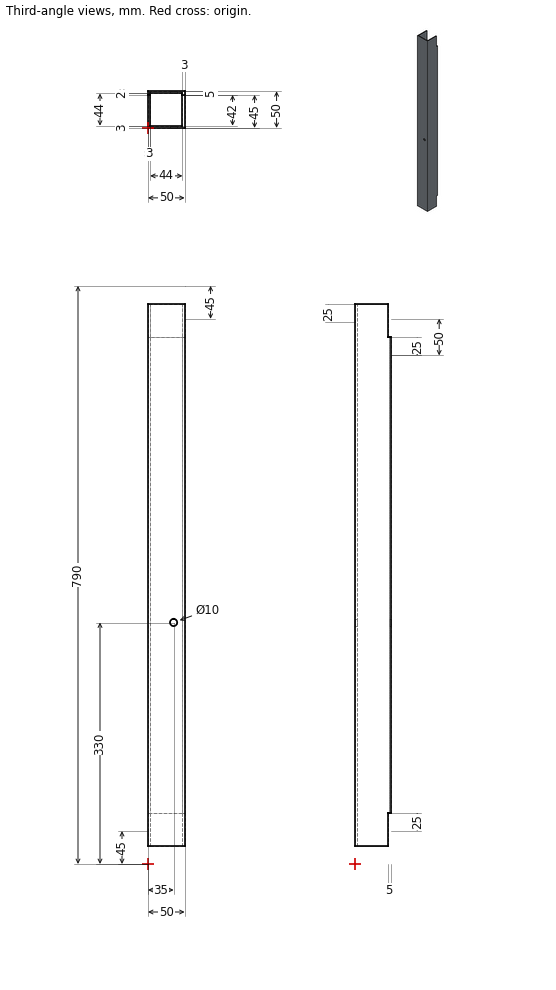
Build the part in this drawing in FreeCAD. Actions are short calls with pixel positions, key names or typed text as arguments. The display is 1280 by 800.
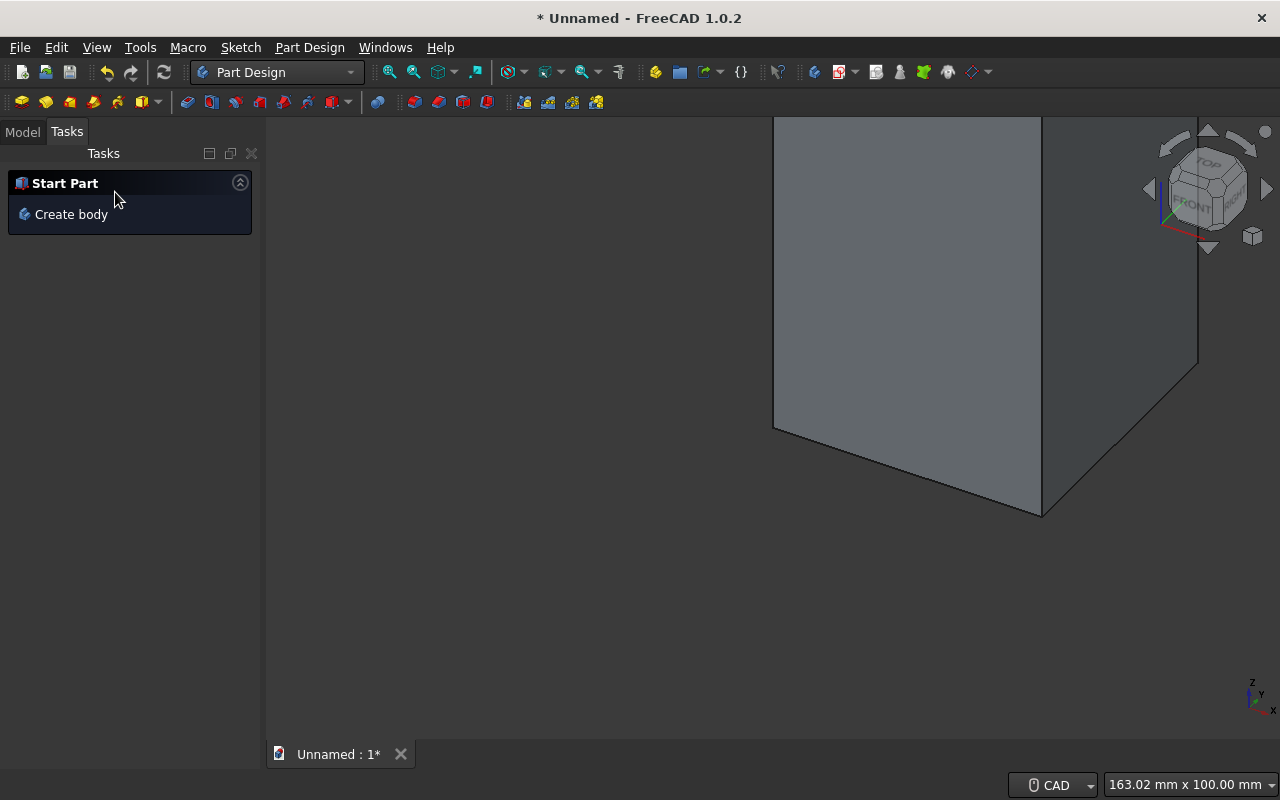
click(390, 72)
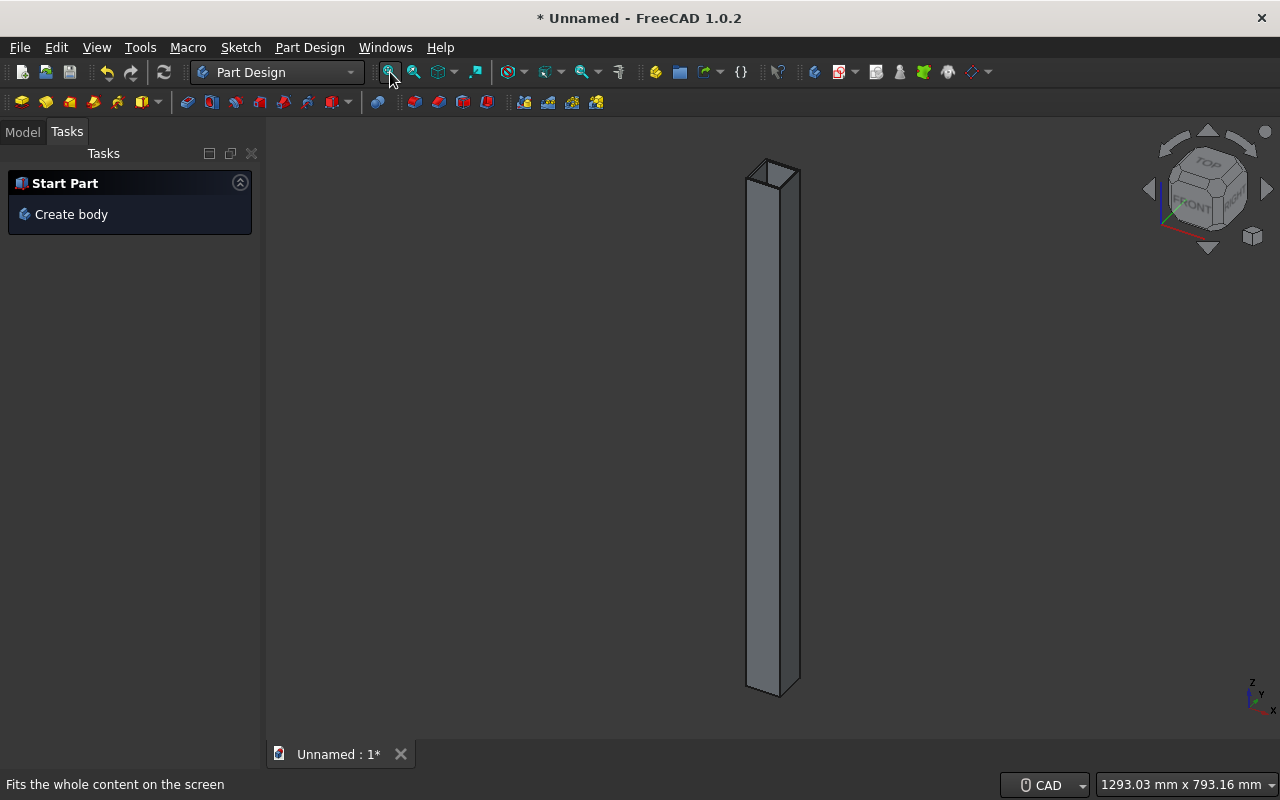
key(4)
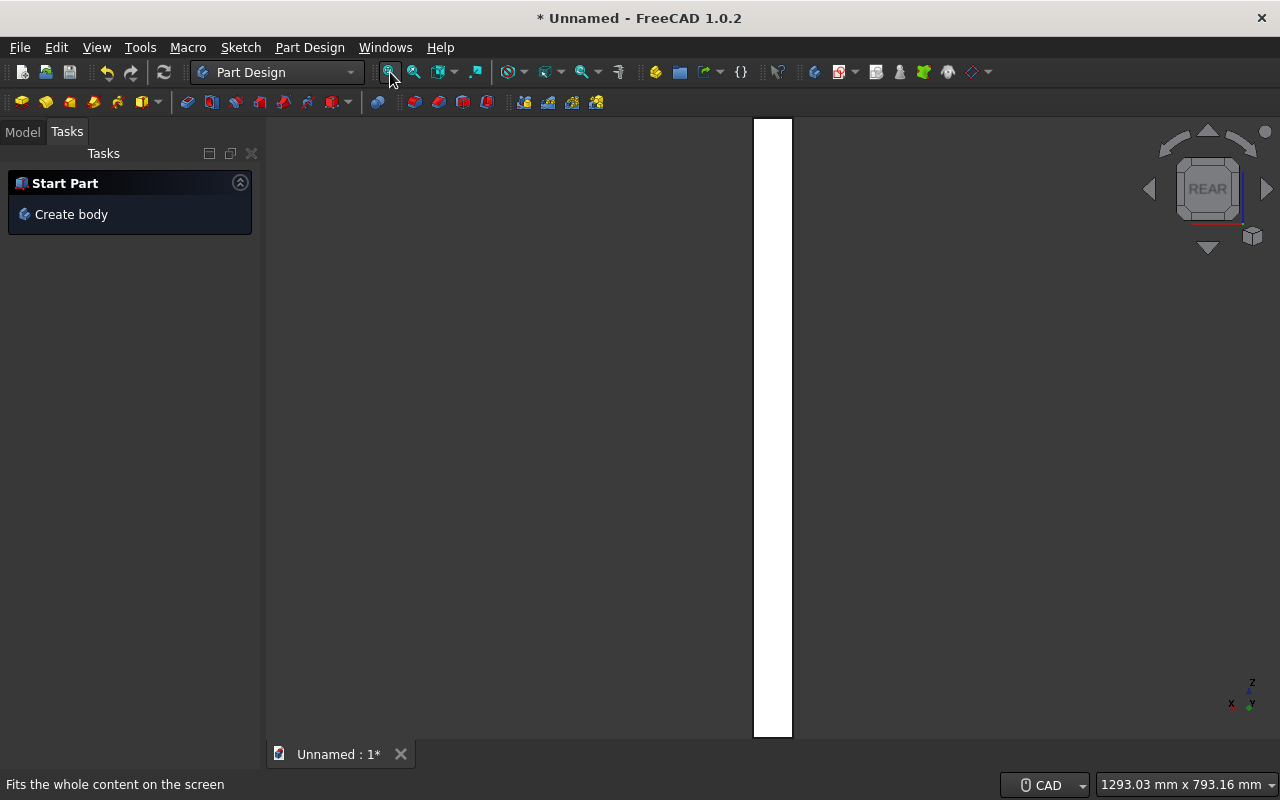
click(773, 161)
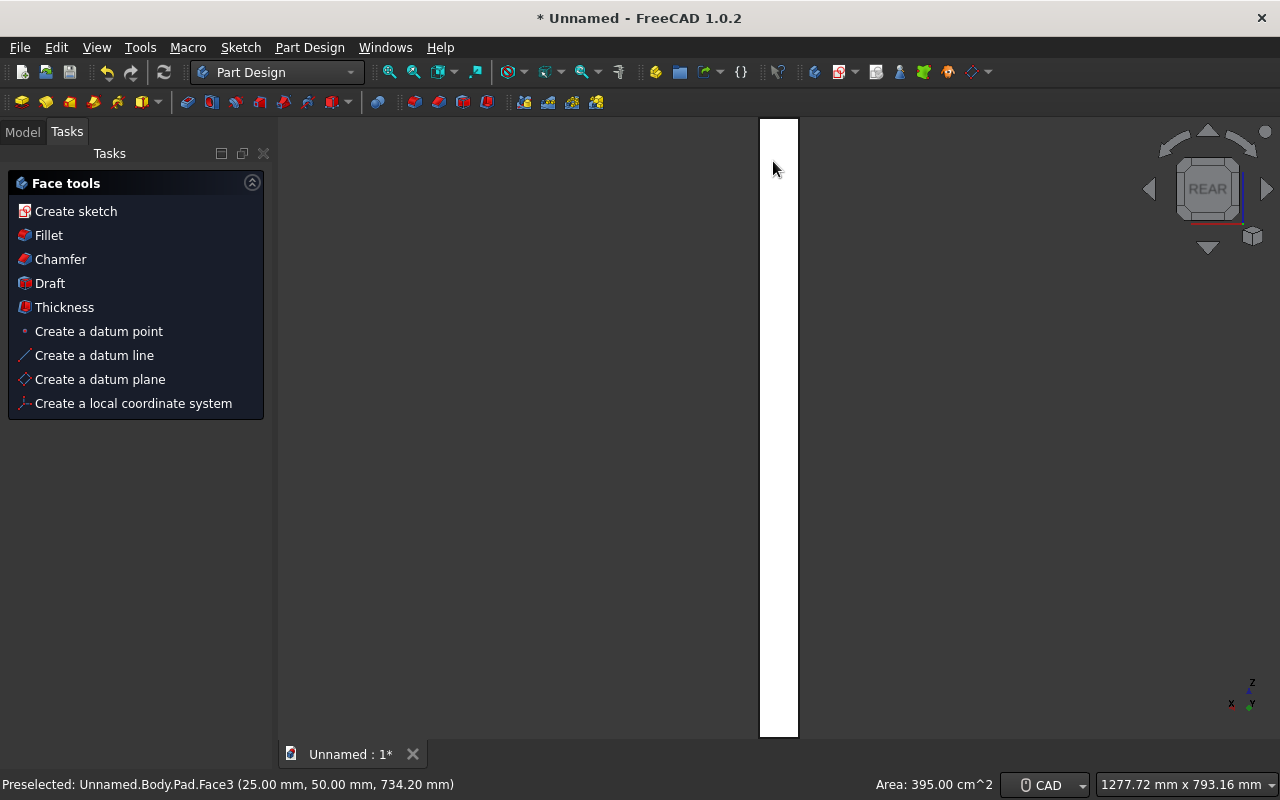
click(840, 72)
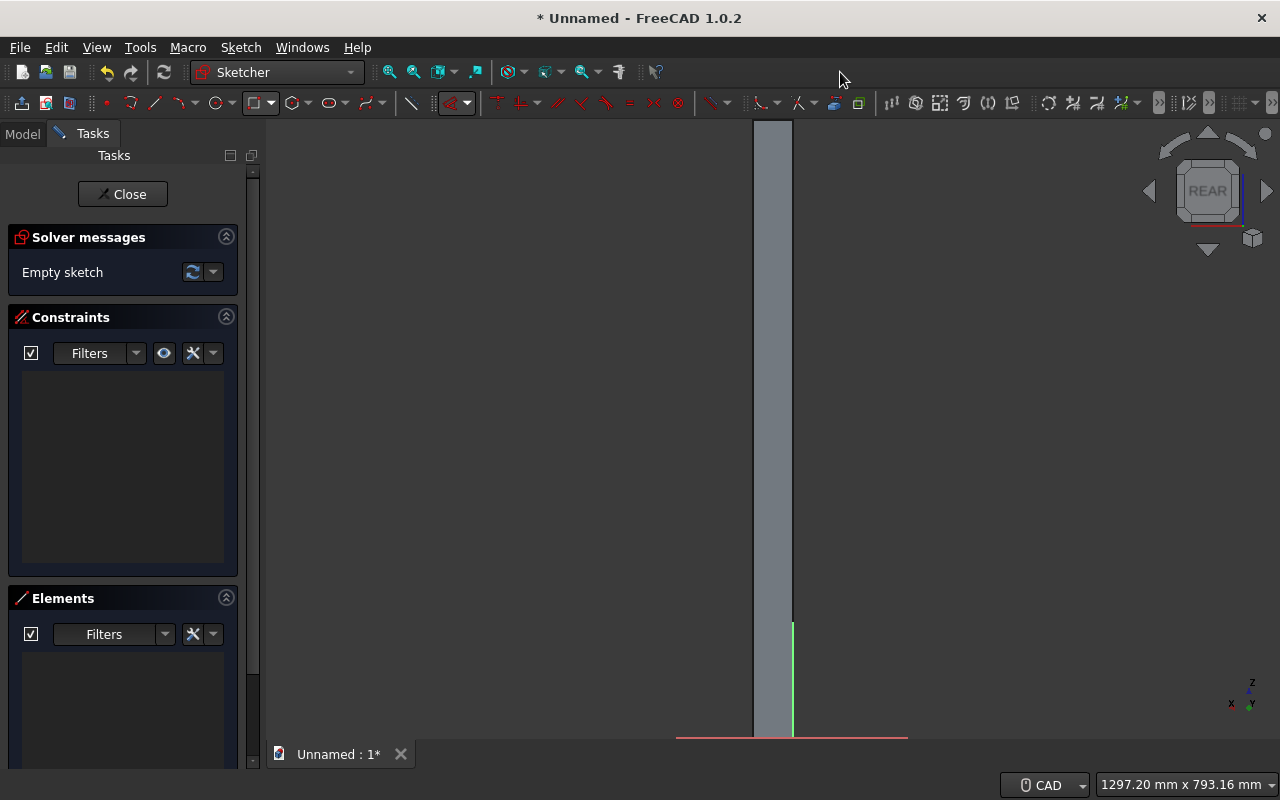
scroll(565, 429, down, 2)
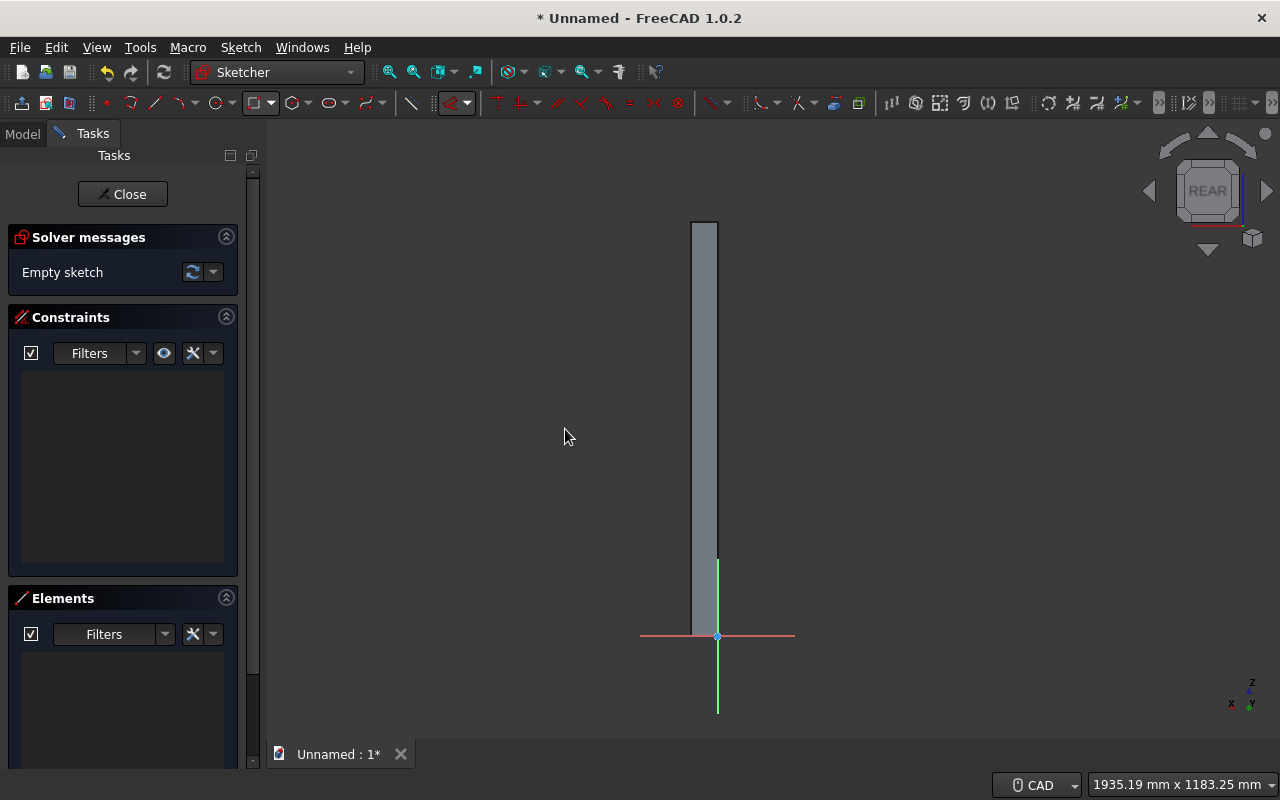
key(g)
key(r)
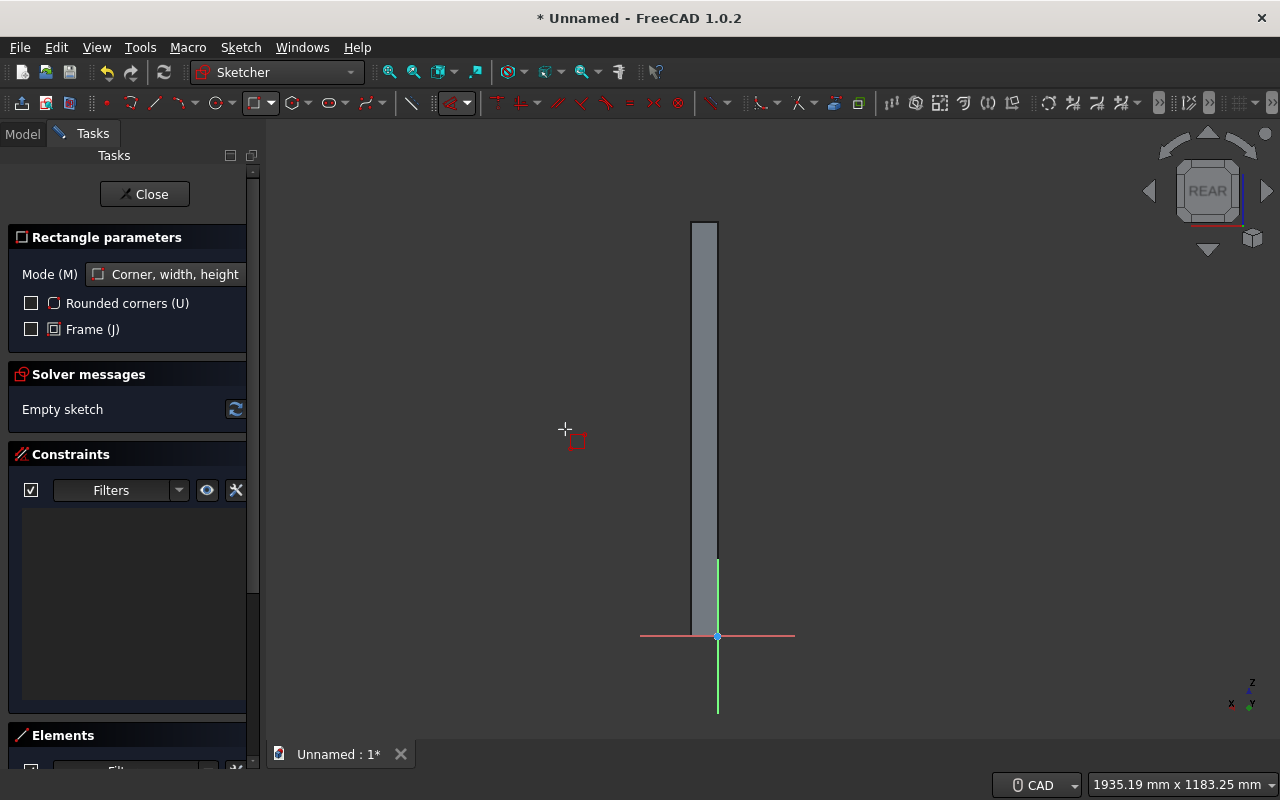
click(718, 636)
click(691, 613)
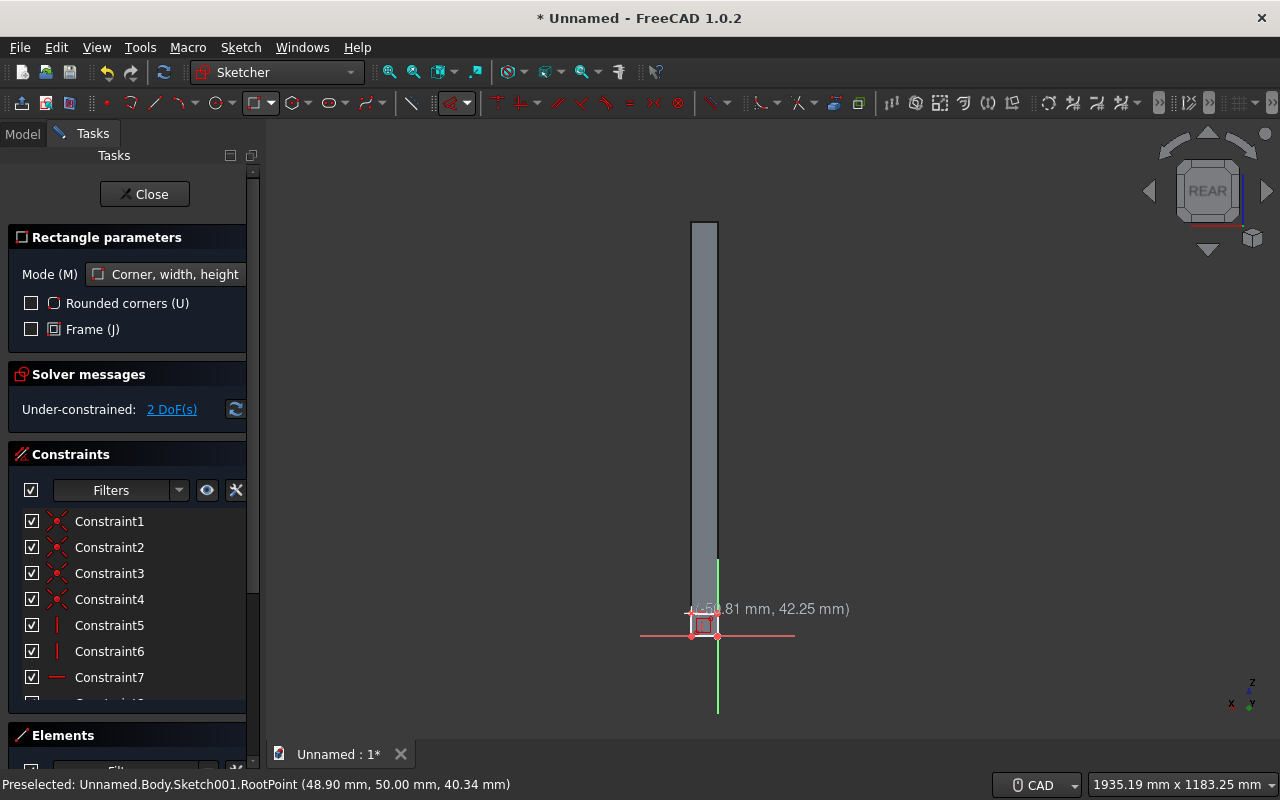
click(691, 222)
click(718, 246)
key(Escape)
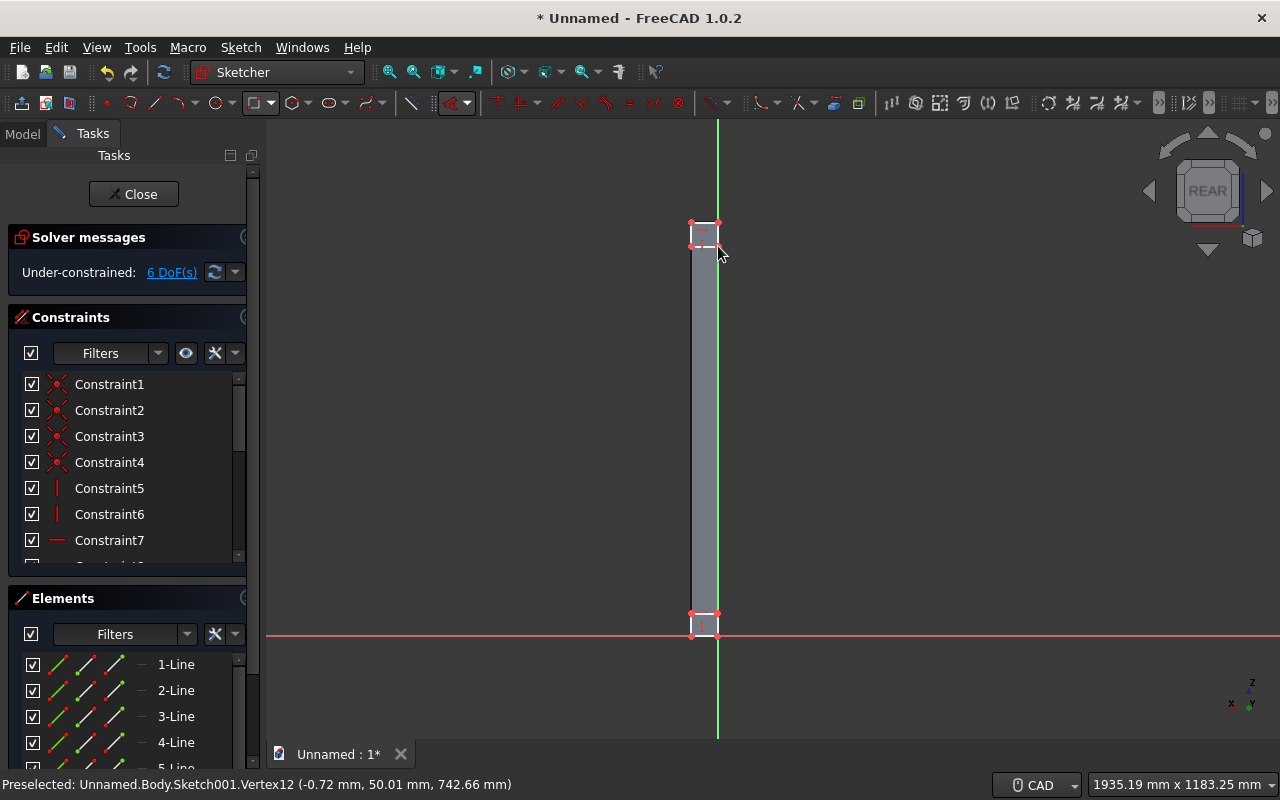
click(718, 247)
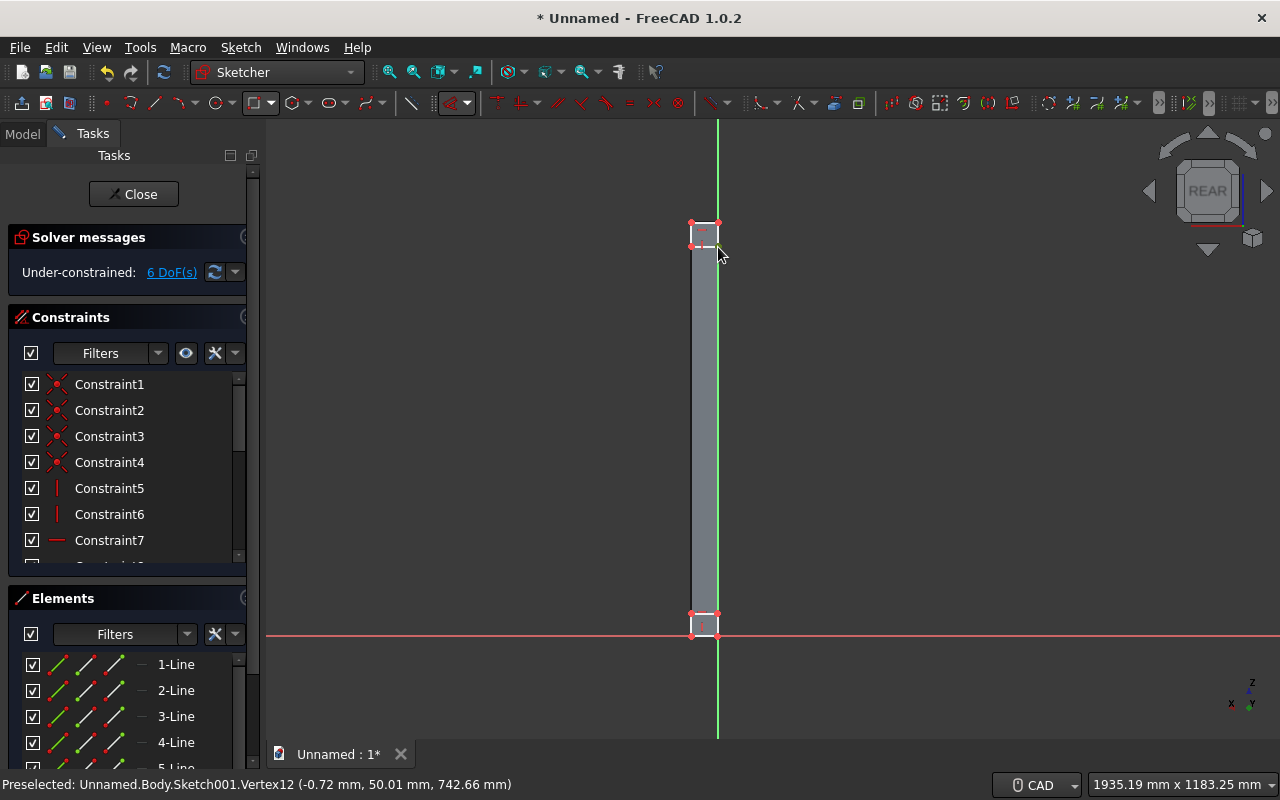
click(718, 671)